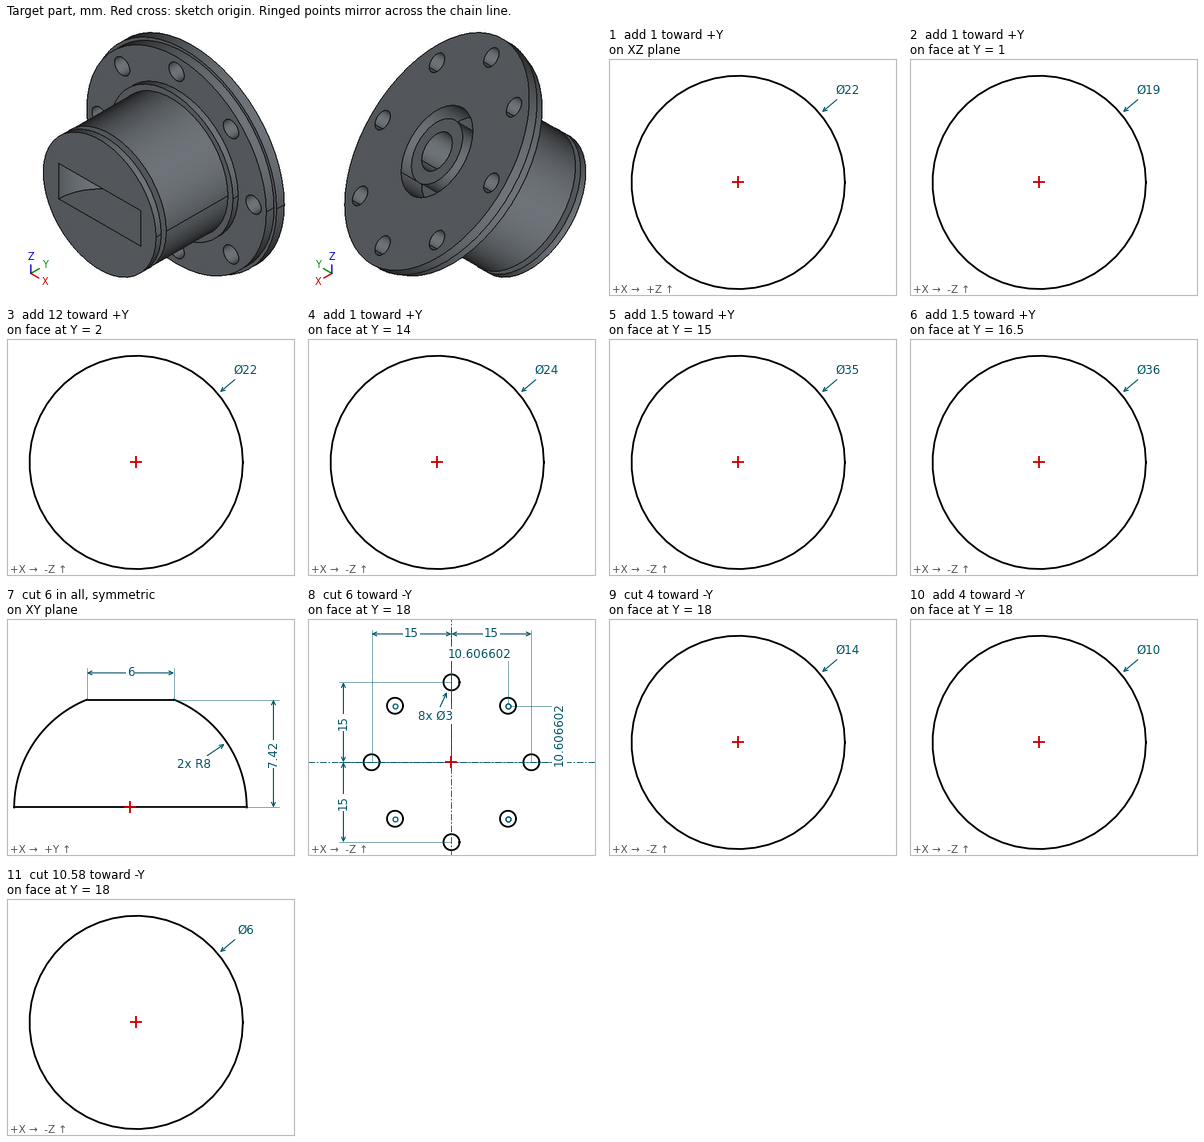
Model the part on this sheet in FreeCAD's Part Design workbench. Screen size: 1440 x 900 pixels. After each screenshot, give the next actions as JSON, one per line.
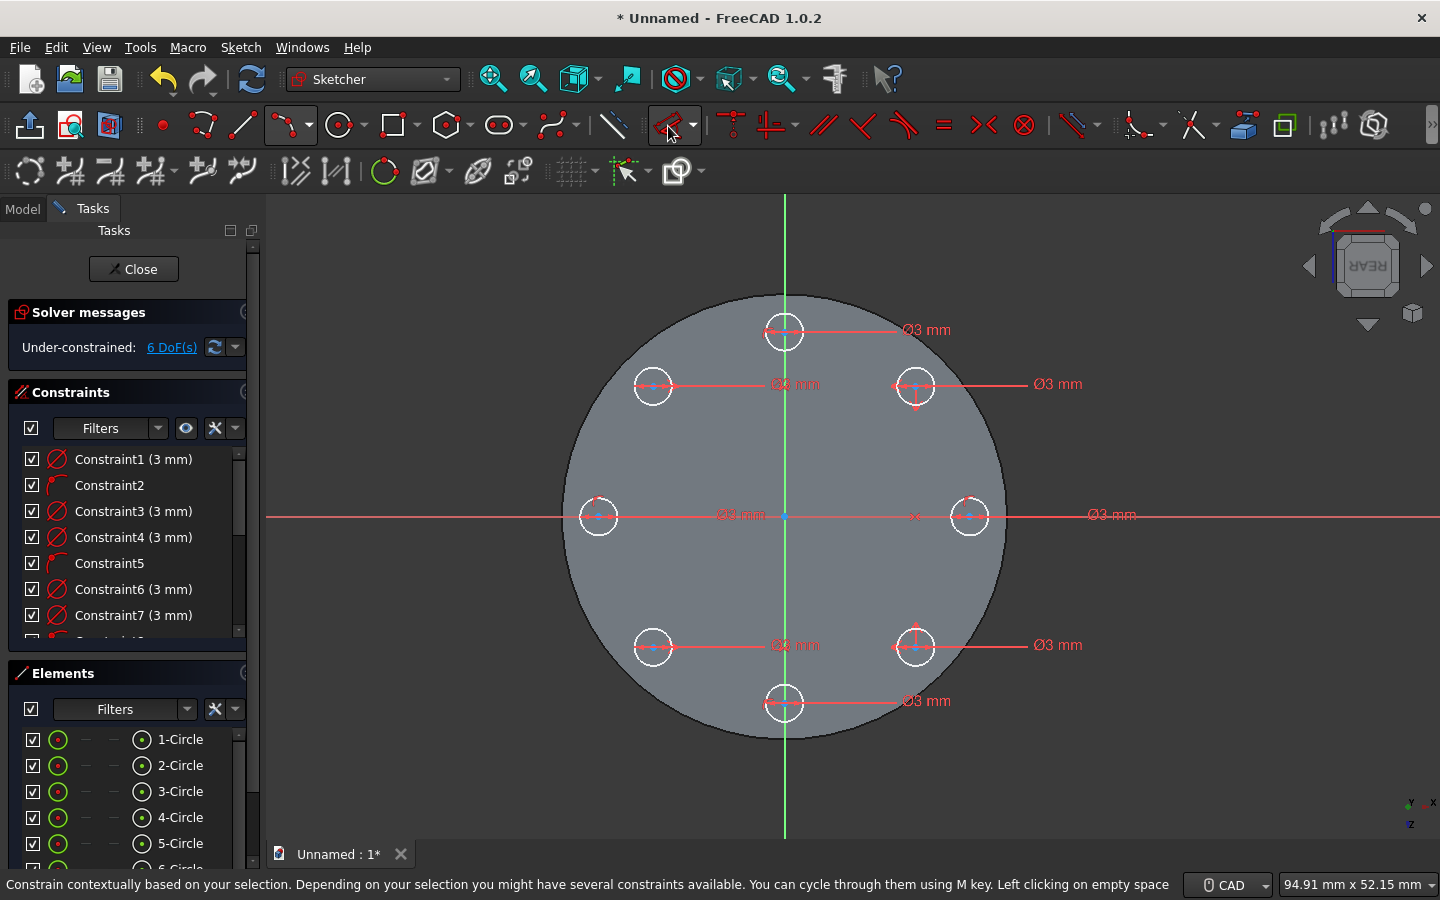
{"action": "left_click", "coordinate": [785, 332]}
{"action": "left_click", "coordinate": [819, 424]}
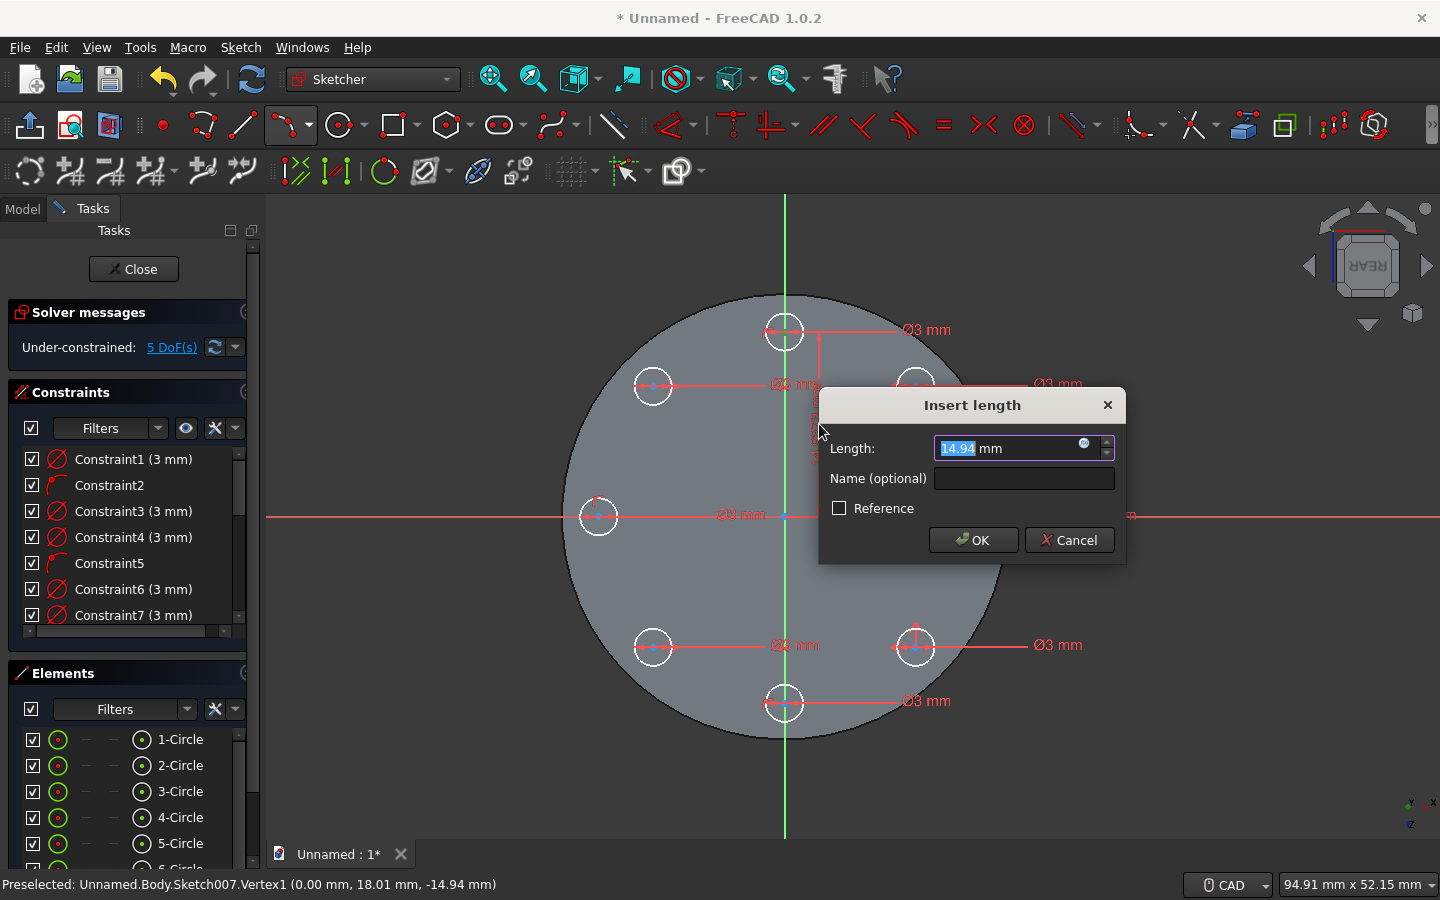
{"action": "type", "text": "15"}
{"action": "key", "text": "Return"}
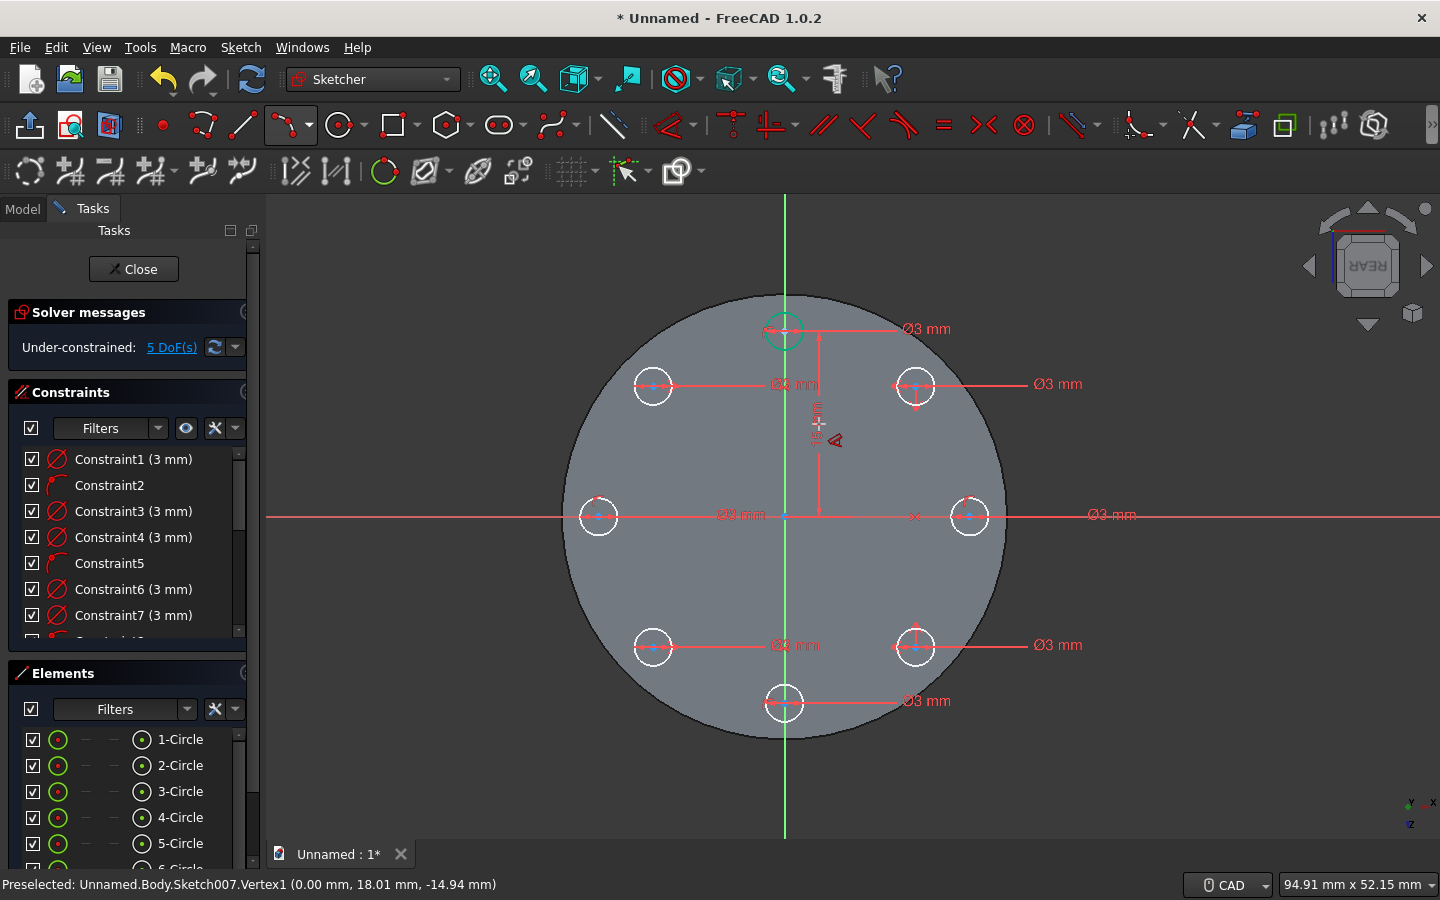
{"action": "left_click", "coordinate": [970, 517]}
{"action": "left_click", "coordinate": [877, 551]}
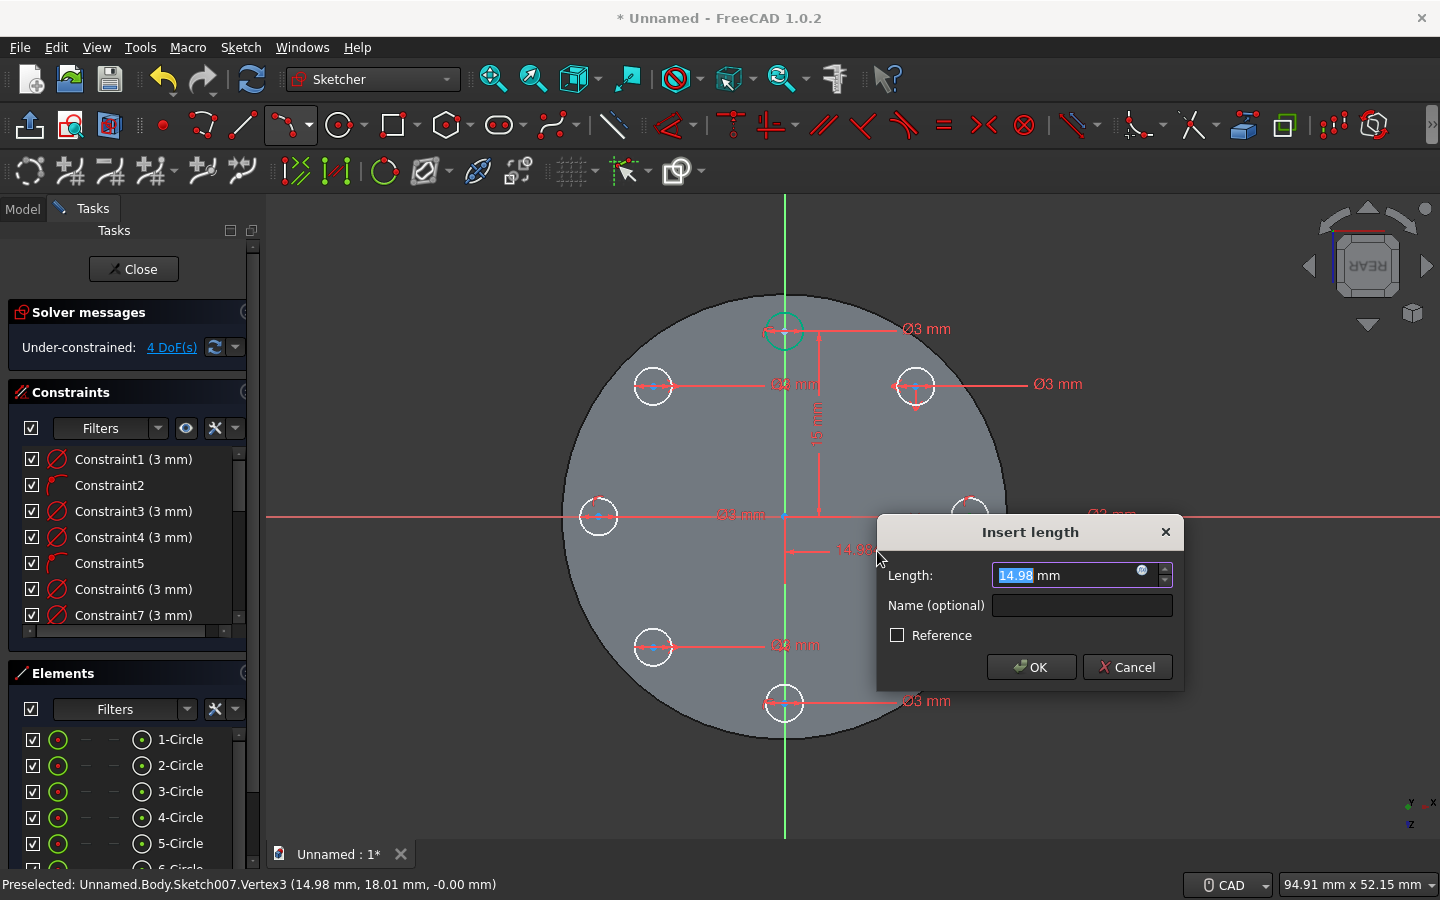
{"action": "type", "text": "15"}
{"action": "key", "text": "Return"}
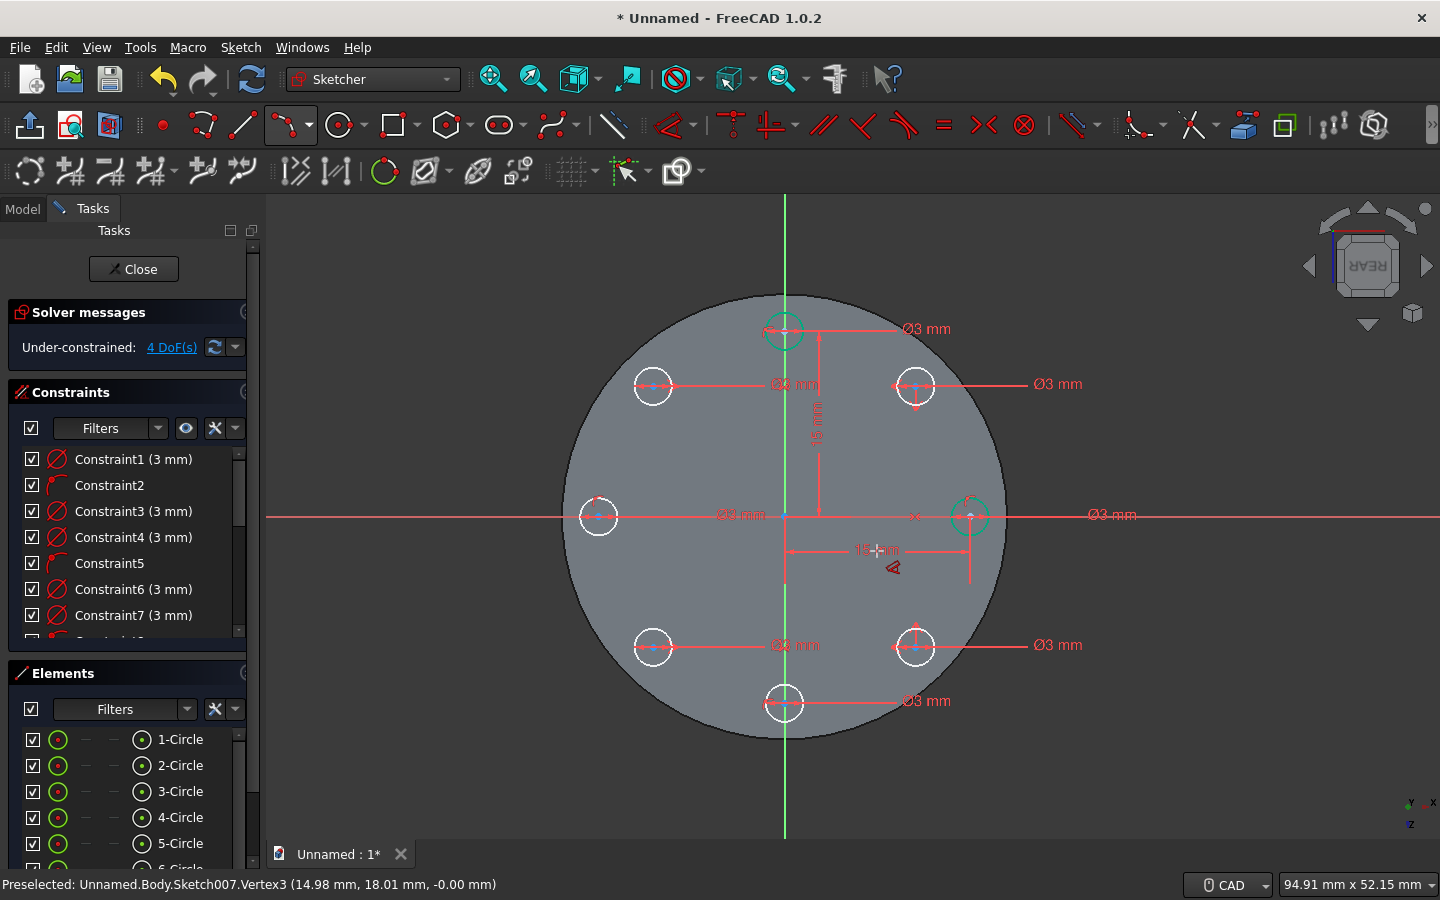
{"action": "left_click", "coordinate": [785, 703]}
{"action": "left_click", "coordinate": [819, 610]}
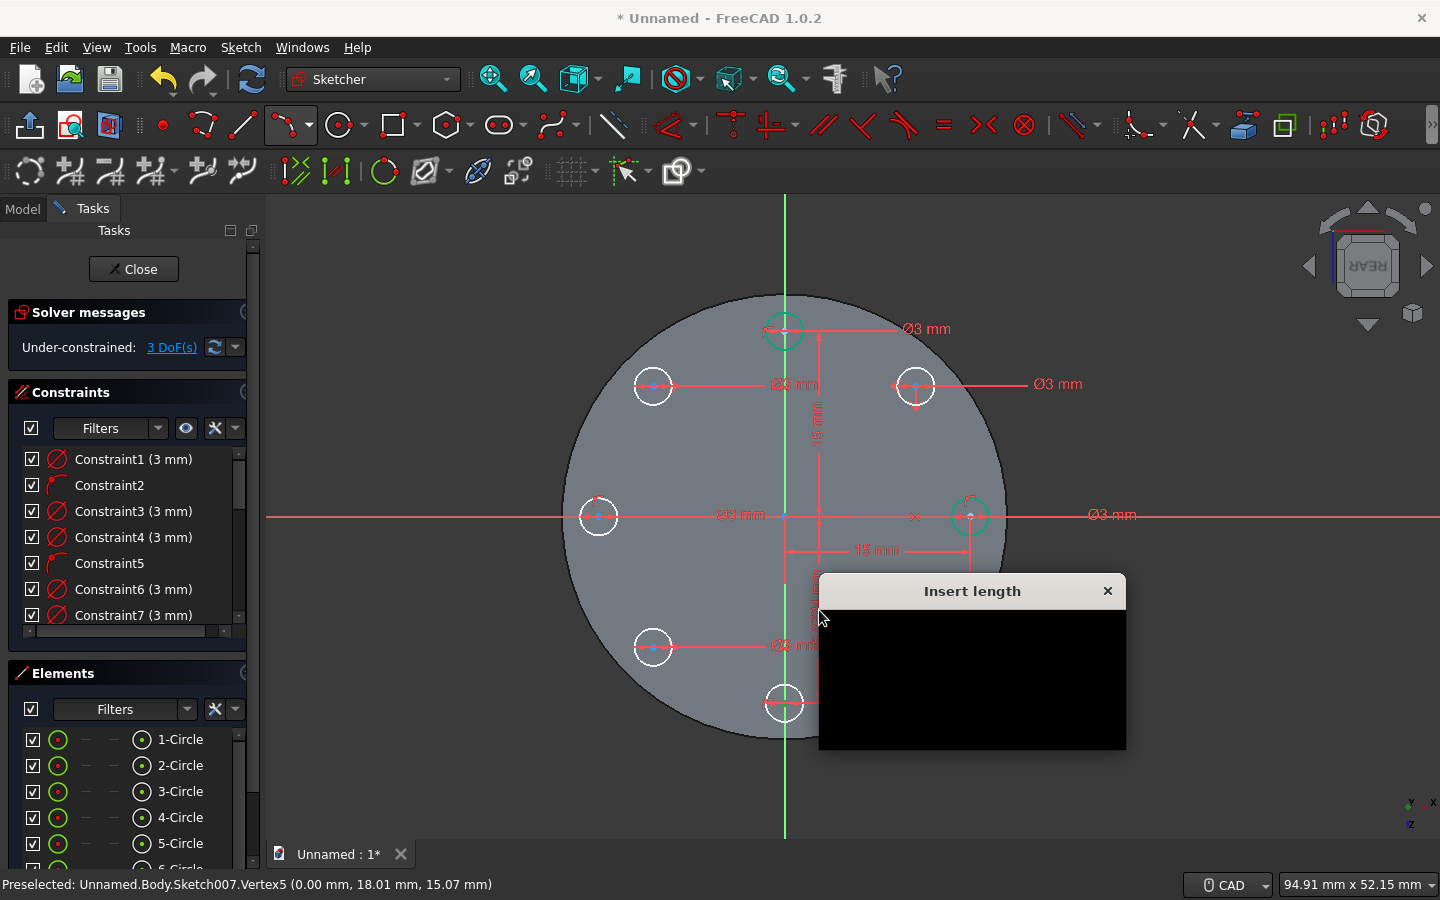
{"action": "type", "text": "15"}
{"action": "key", "text": "Return"}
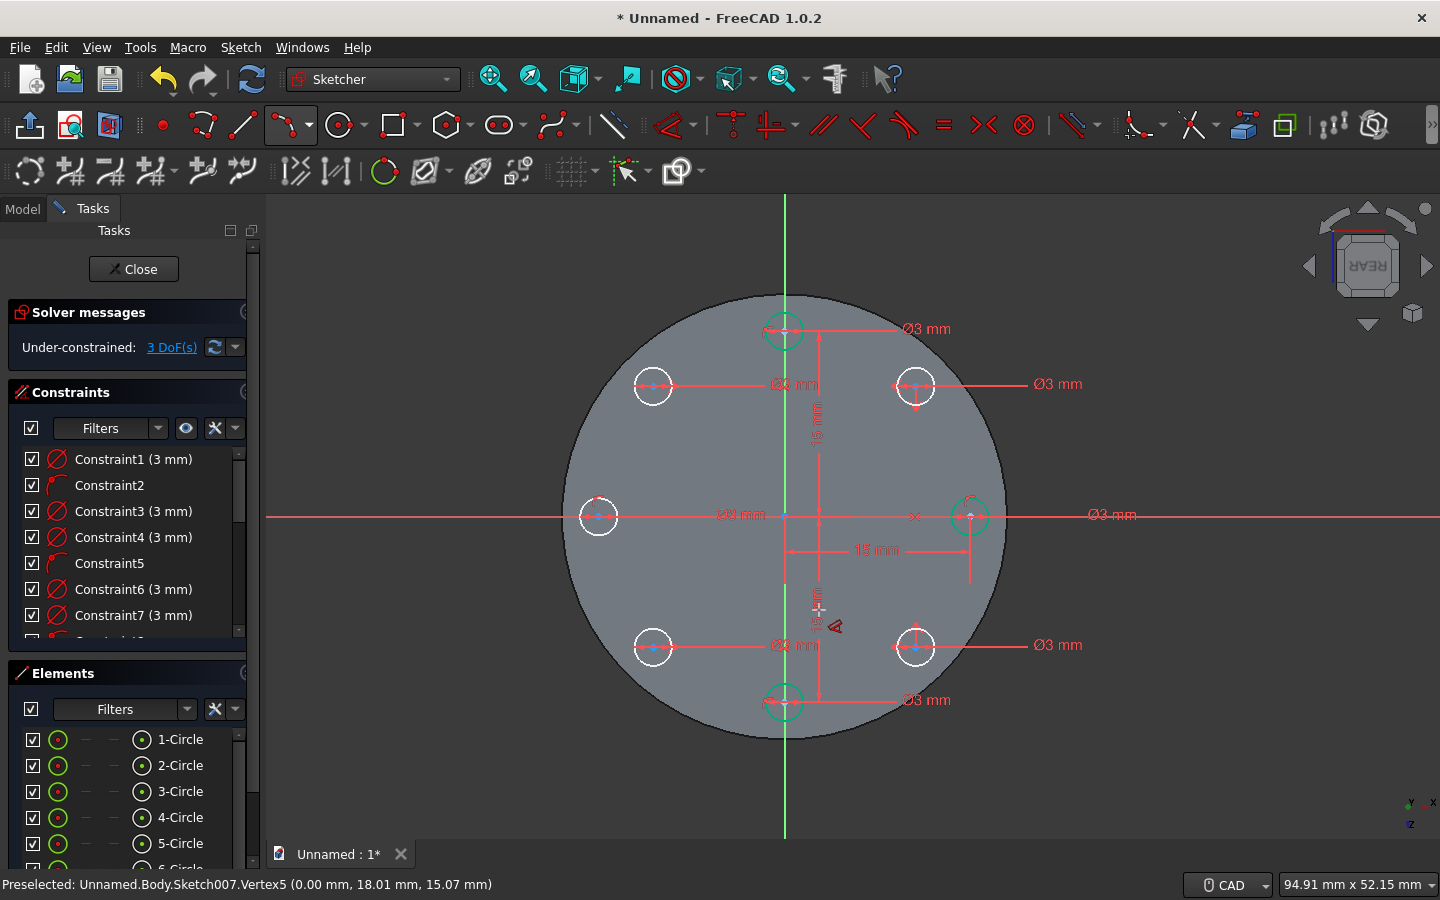
{"action": "left_click", "coordinate": [599, 517]}
{"action": "left_click", "coordinate": [692, 551]}